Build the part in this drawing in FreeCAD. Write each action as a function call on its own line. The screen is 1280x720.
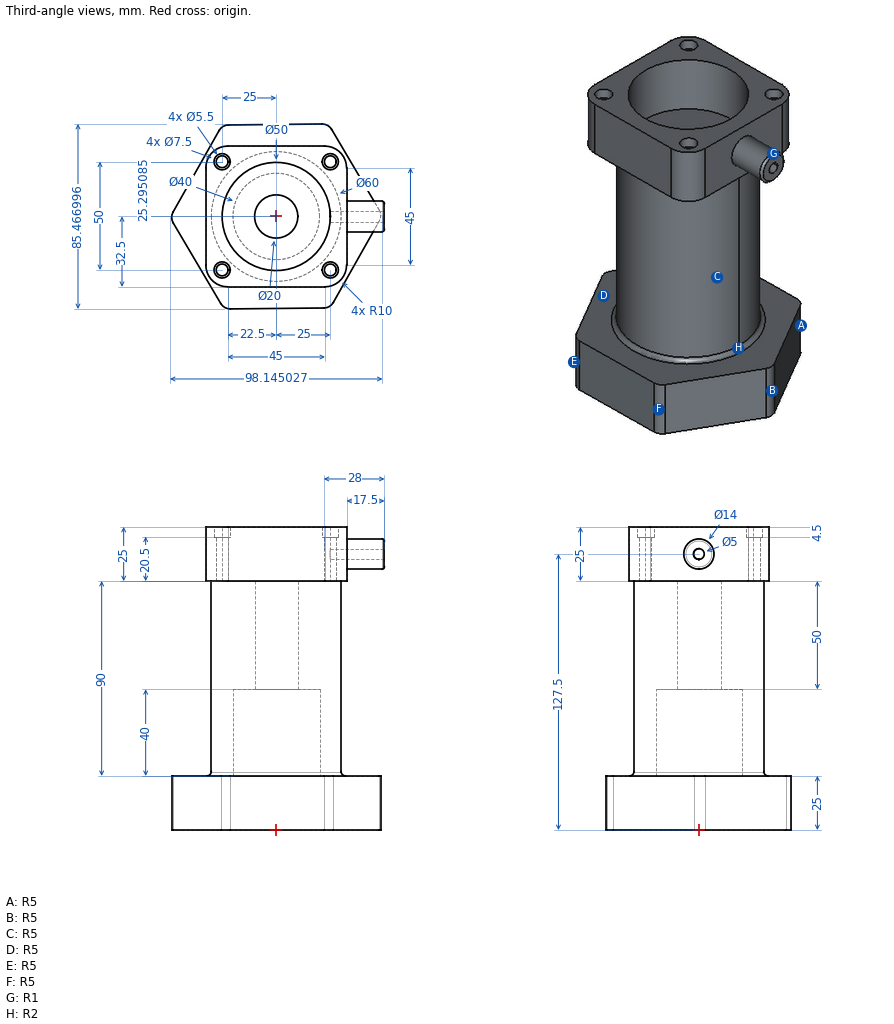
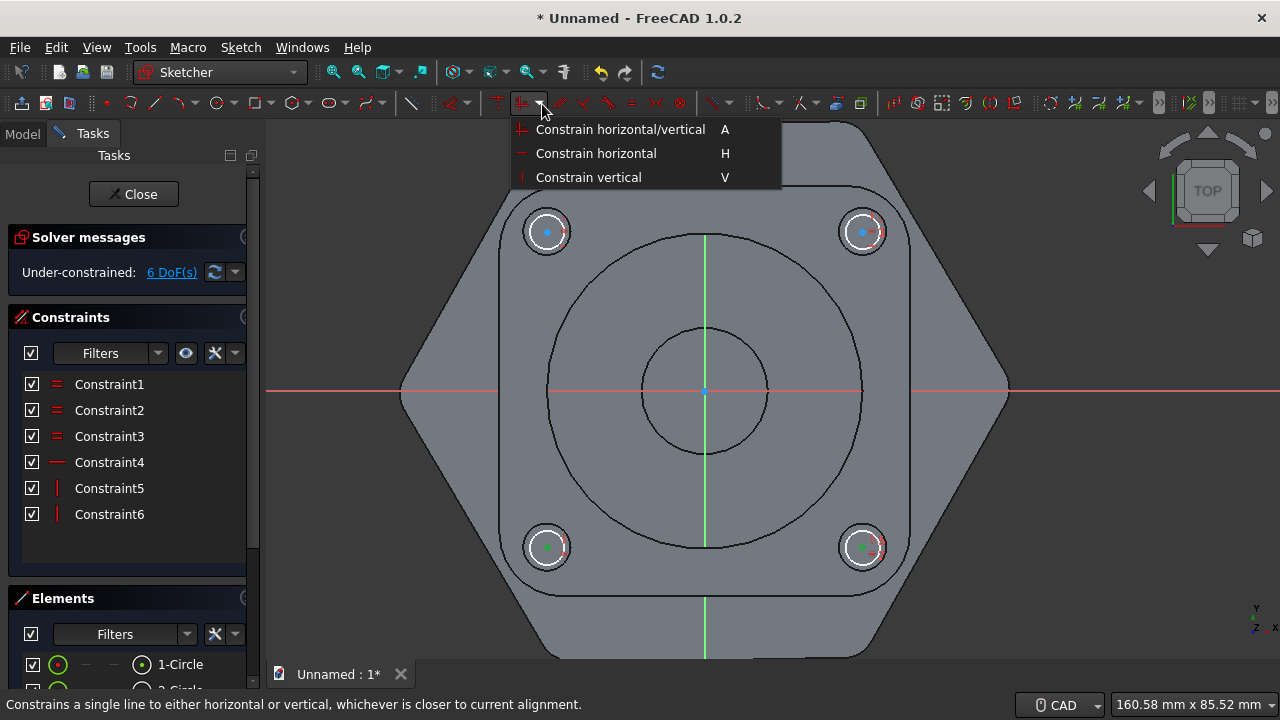
click(646, 153)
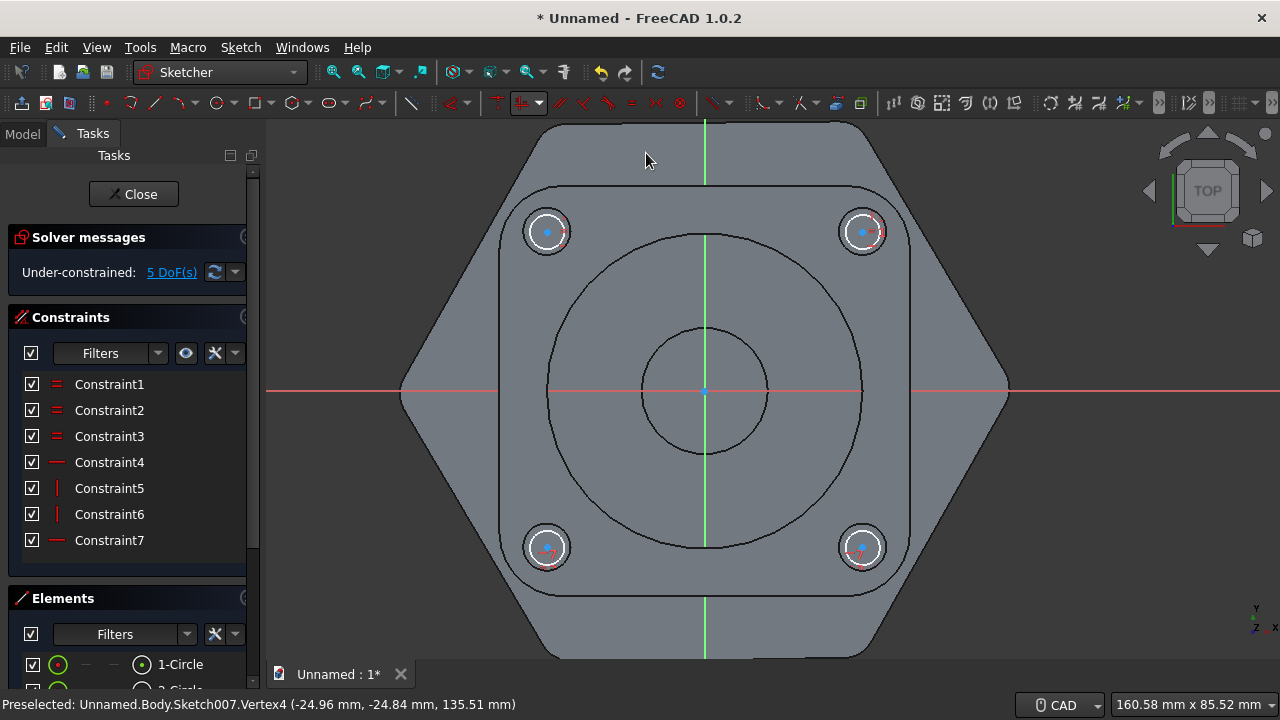
click(450, 104)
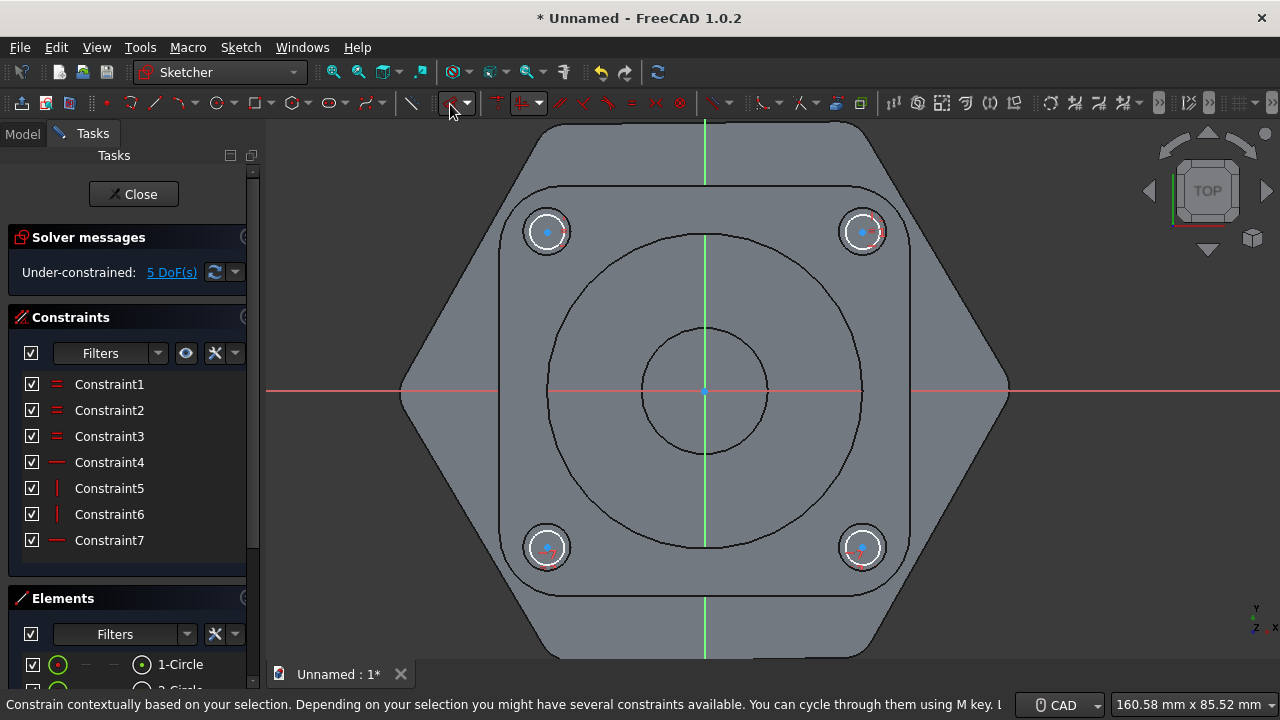
click(559, 220)
click(581, 197)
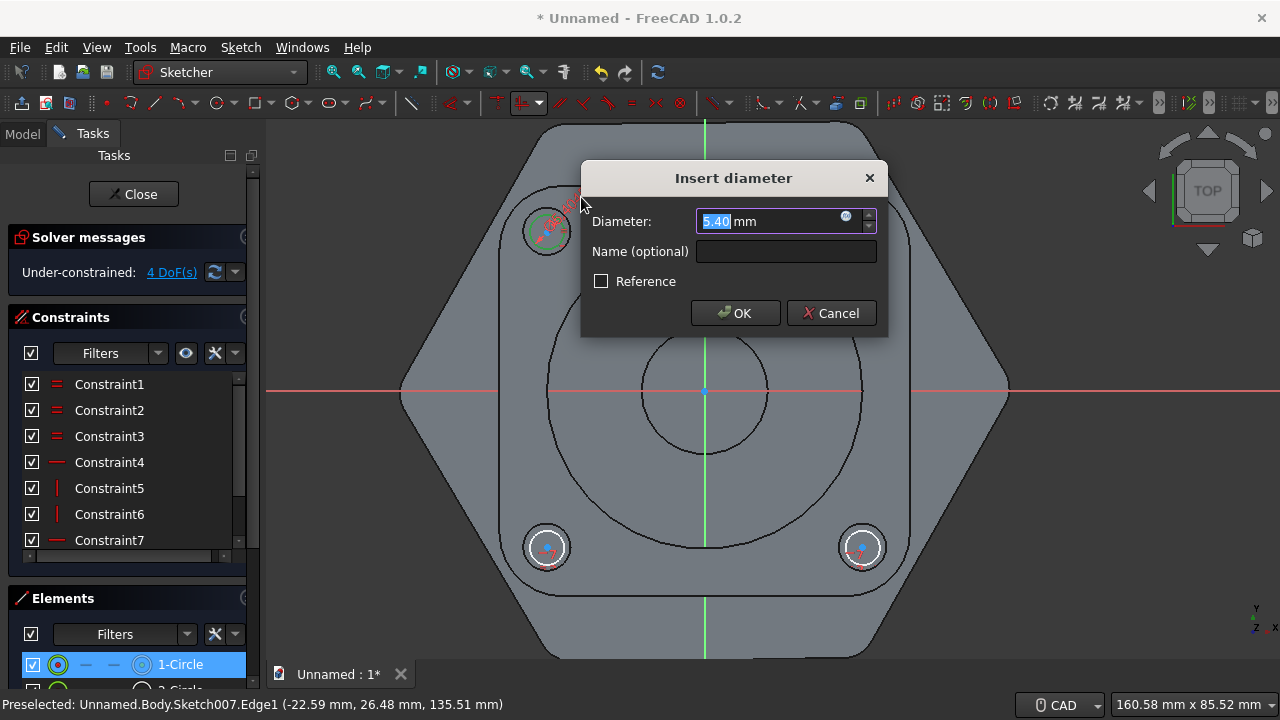
text(5.5)
key(Return)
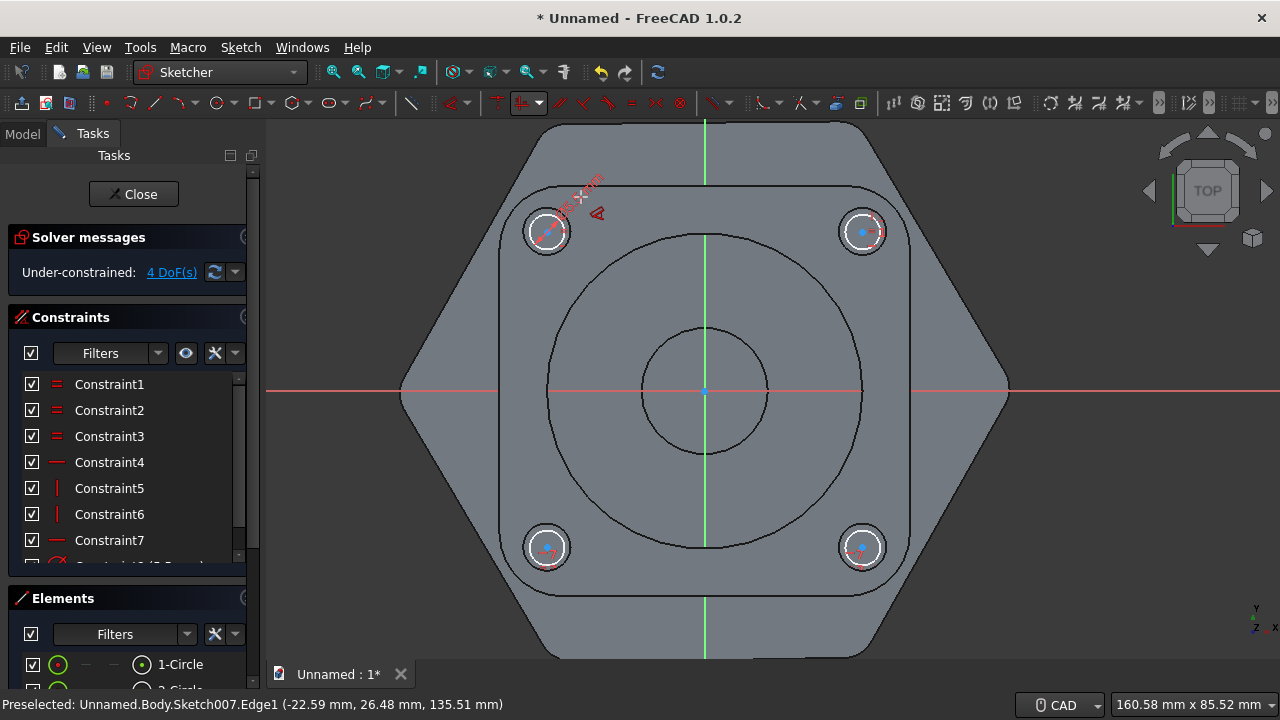
click(547, 232)
click(662, 198)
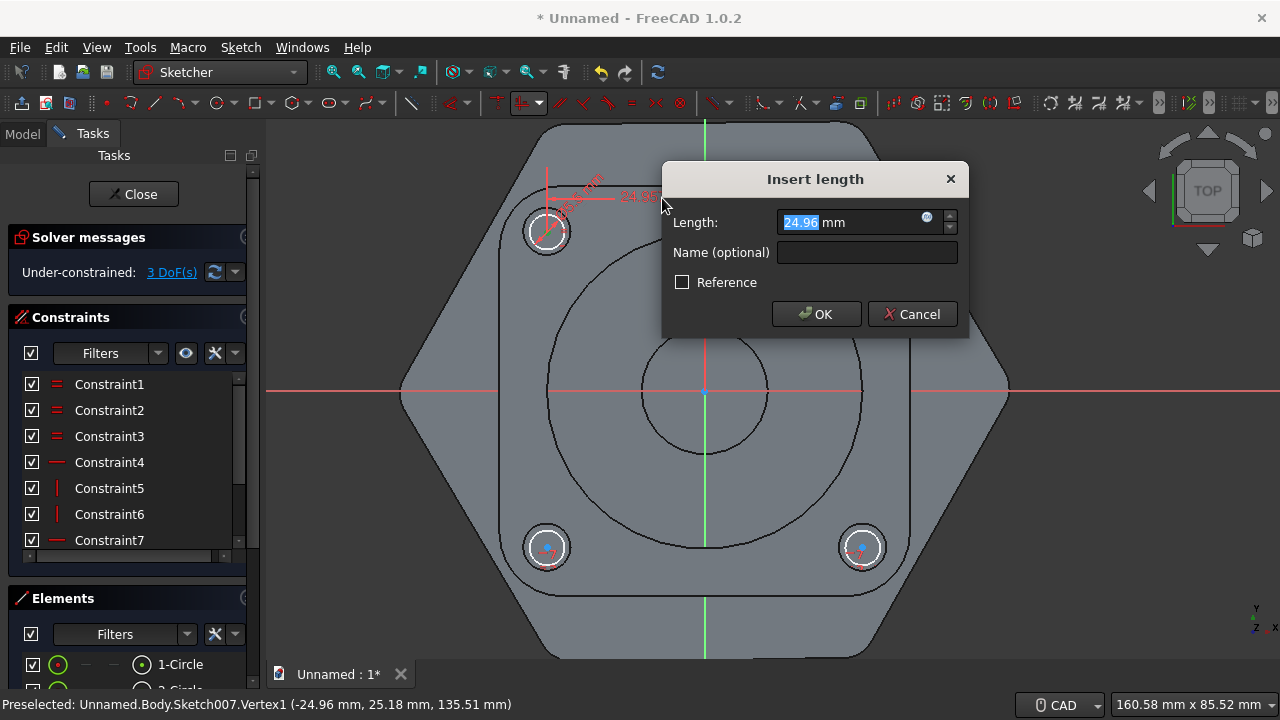
text(25)
key(Return)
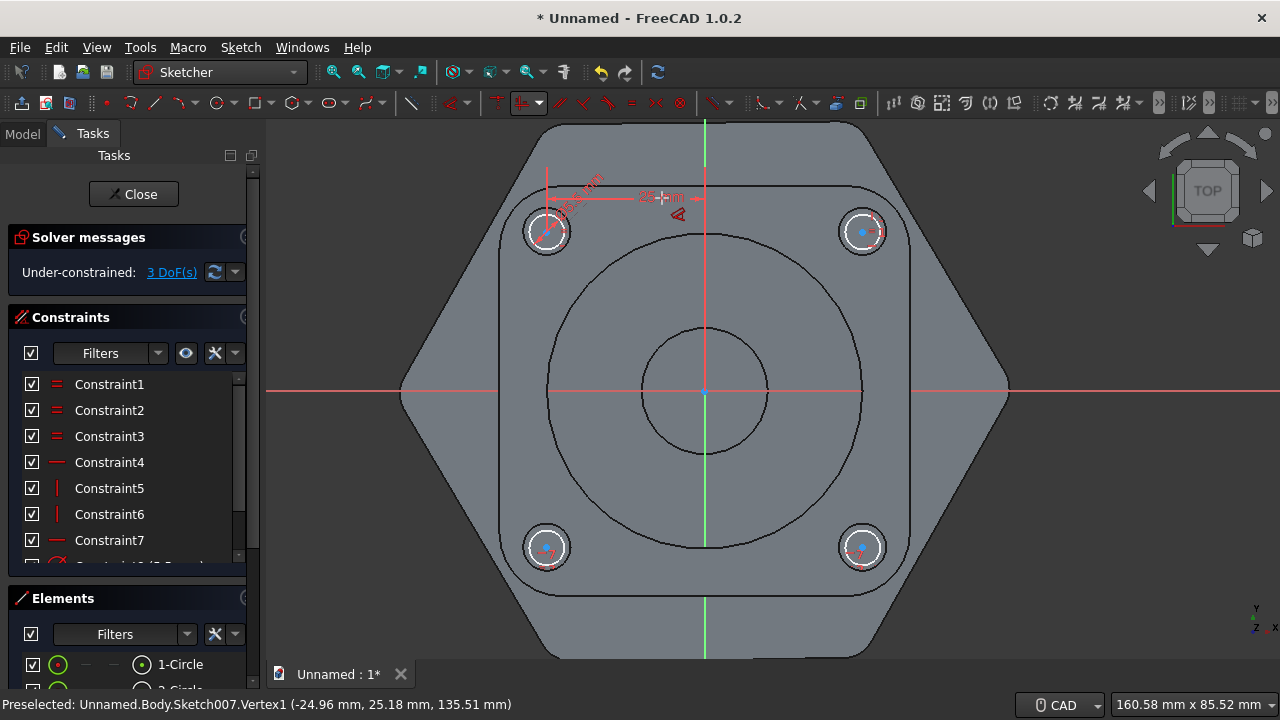
click(863, 232)
click(784, 198)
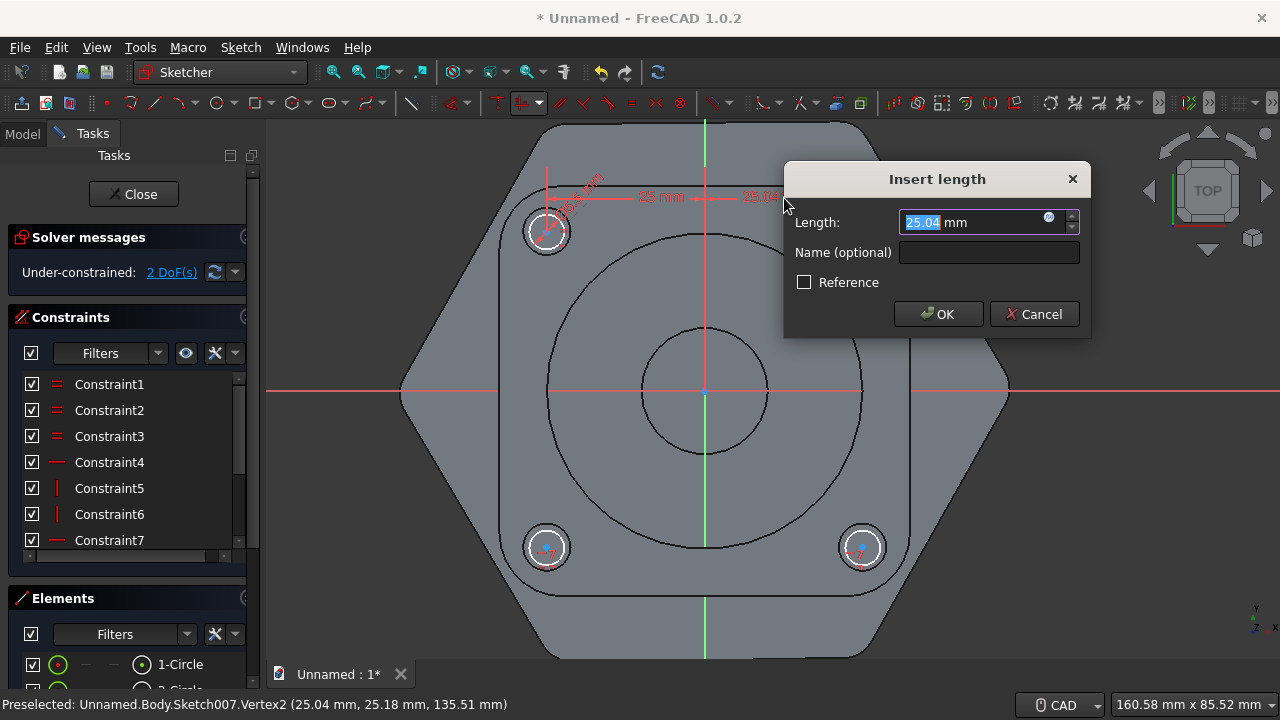
text(25)
key(Return)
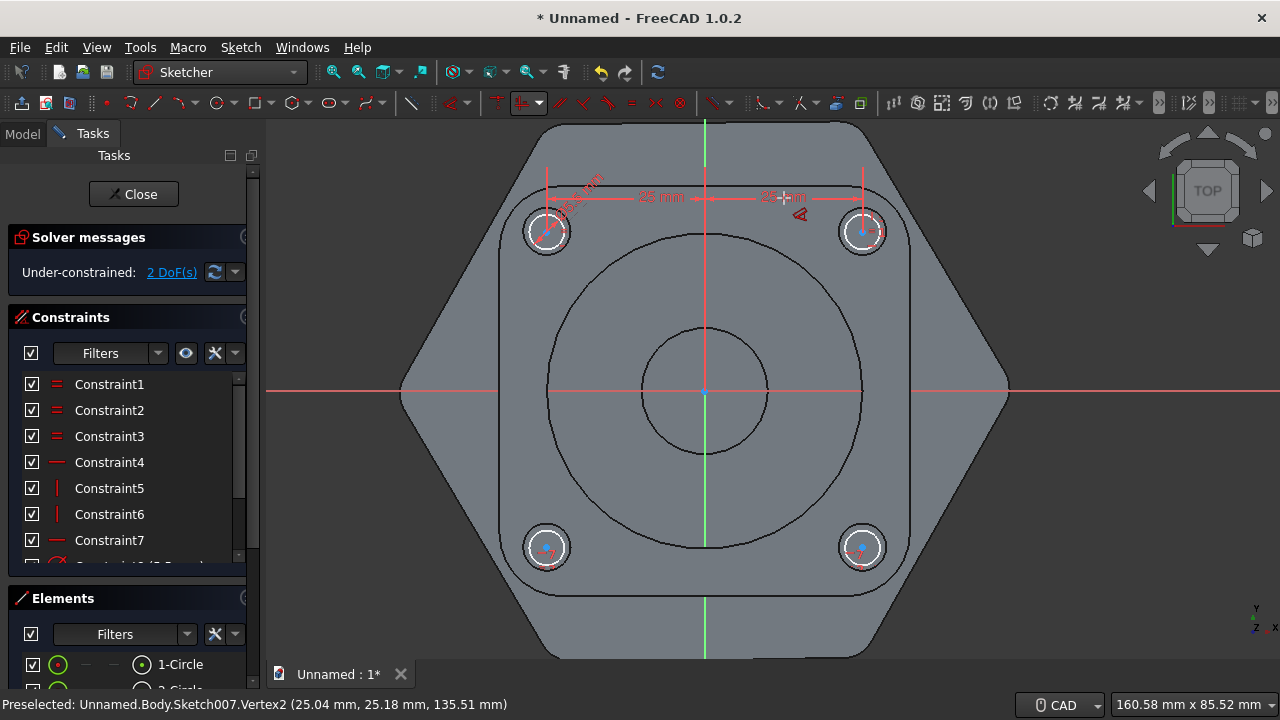
click(863, 232)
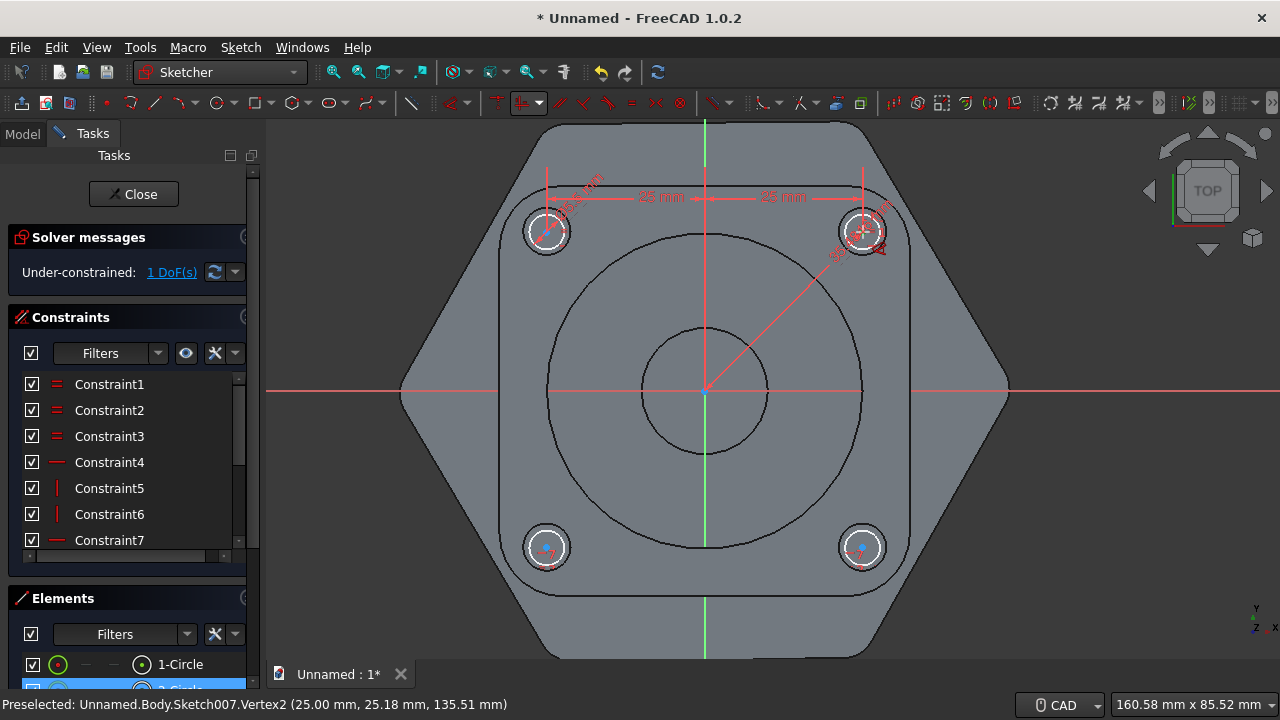
click(863, 548)
click(897, 317)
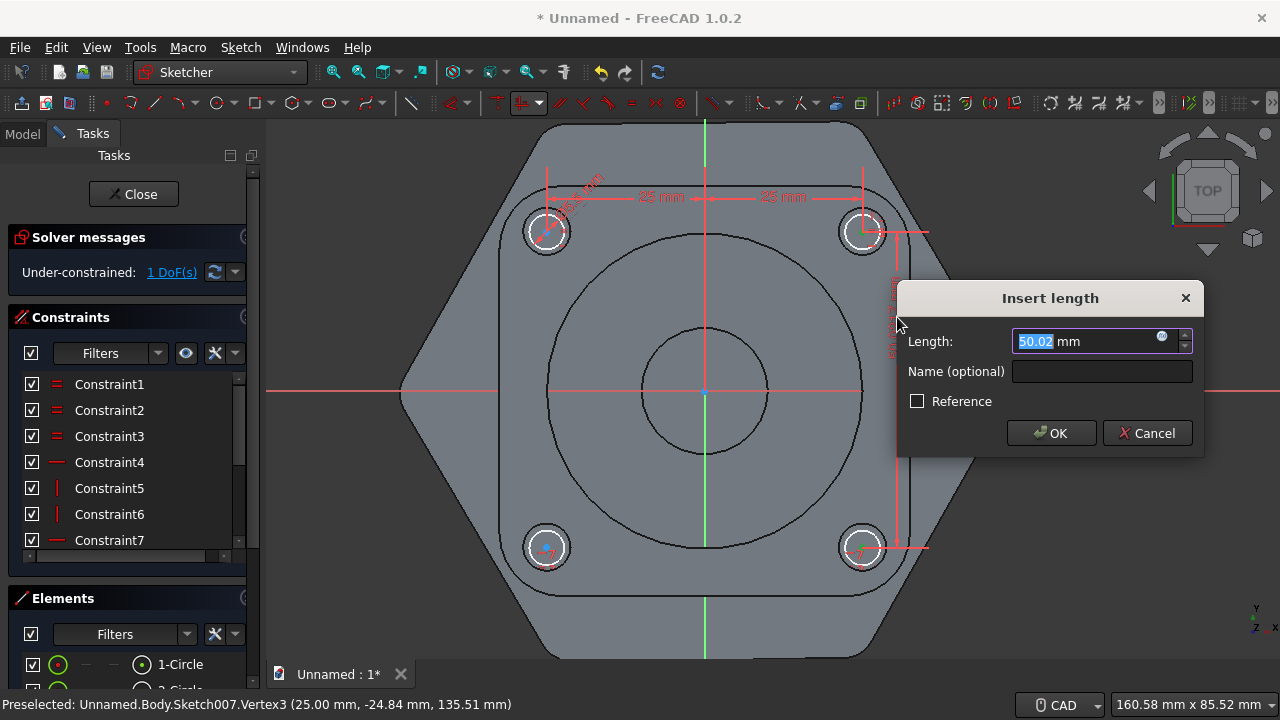
text(50)
key(Return)